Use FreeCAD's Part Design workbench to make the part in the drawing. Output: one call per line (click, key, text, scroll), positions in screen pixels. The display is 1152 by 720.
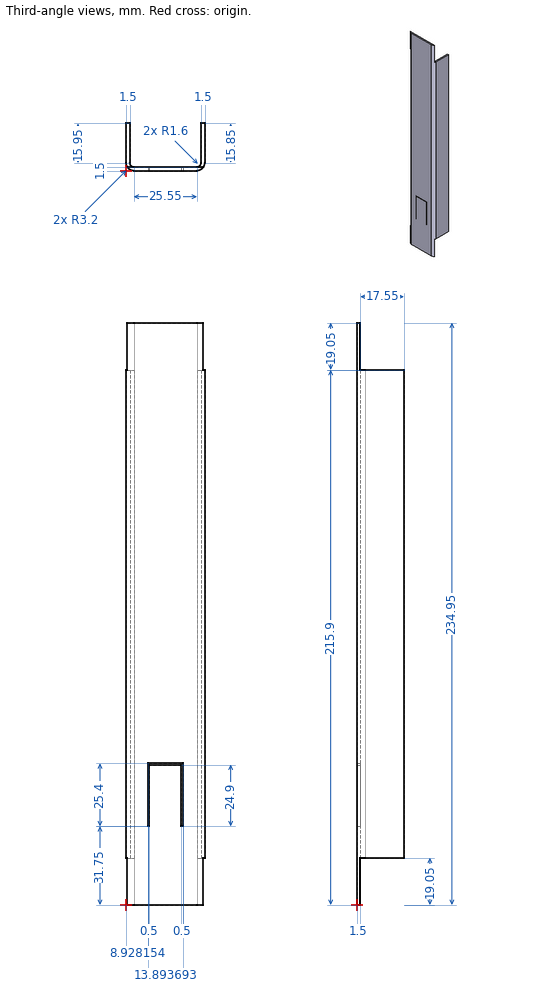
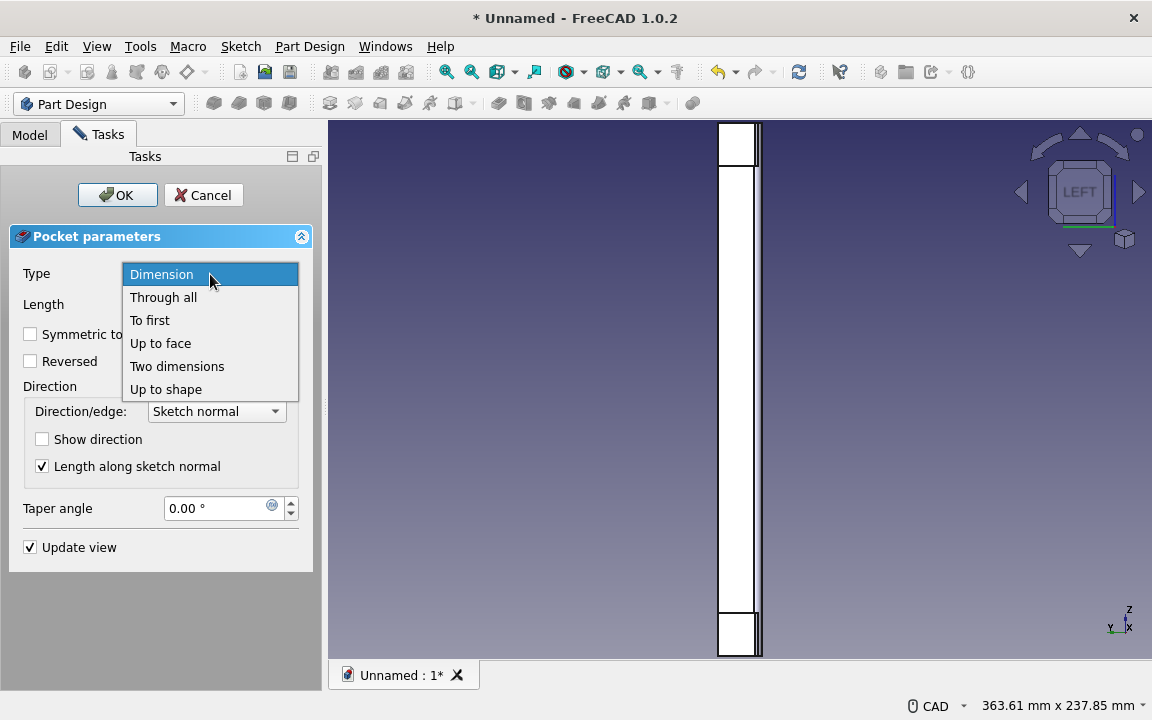
click(208, 298)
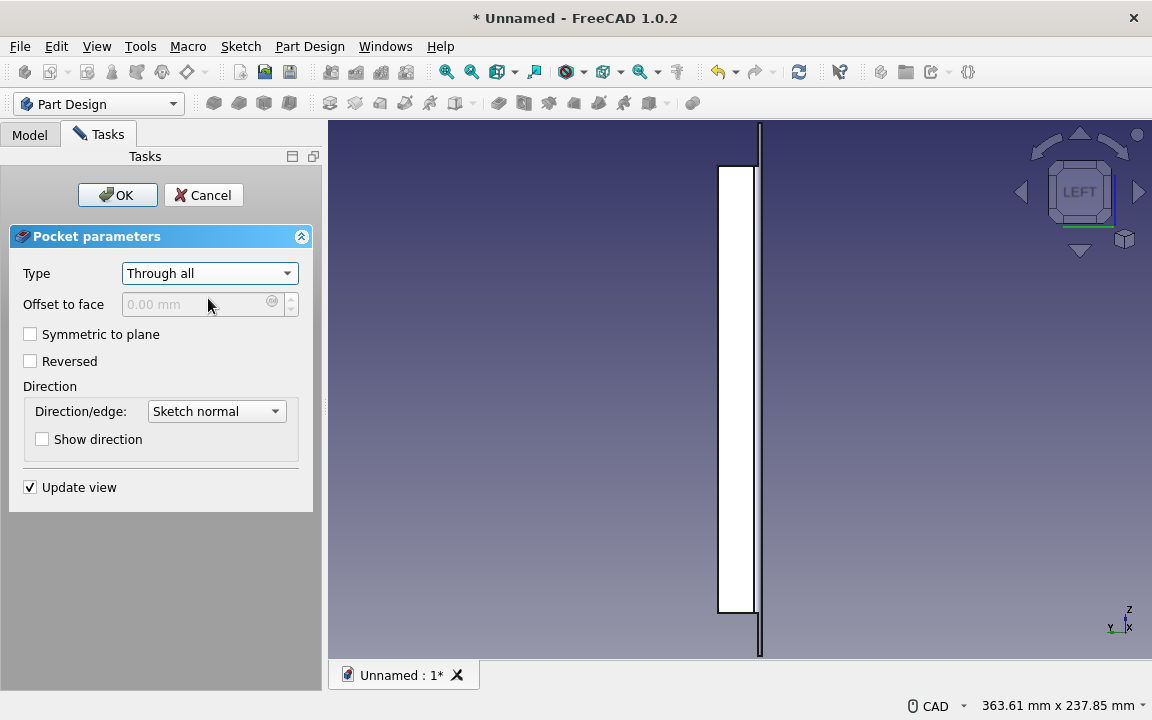
click(118, 195)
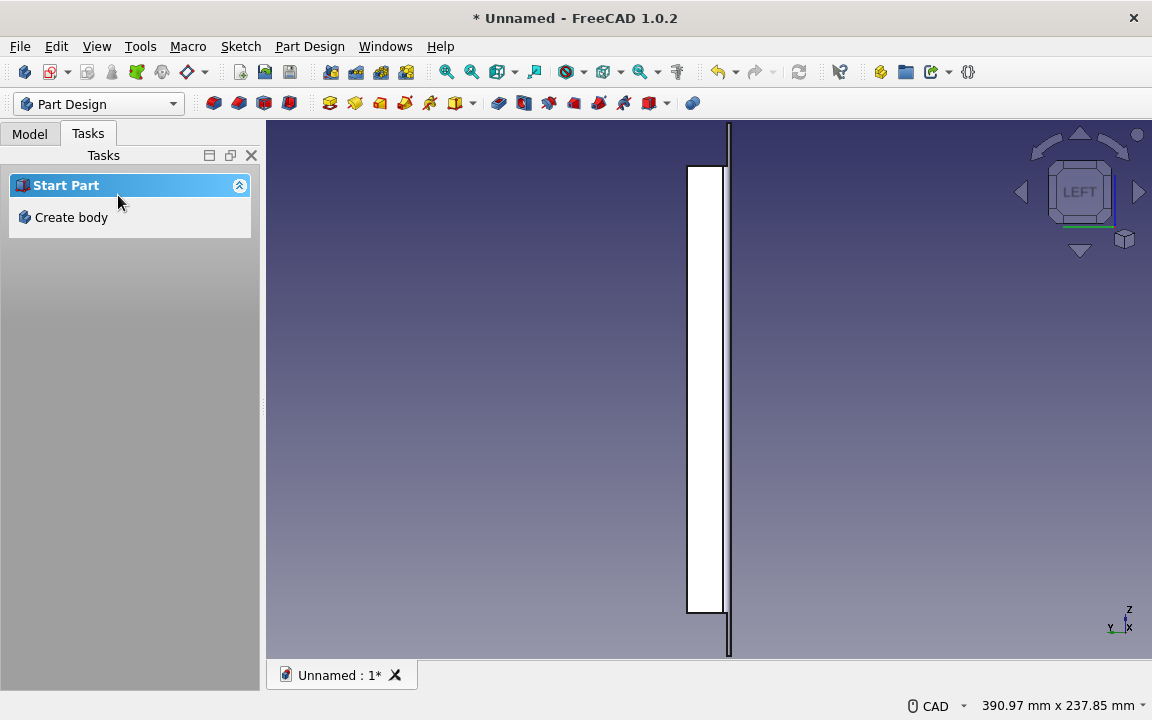
key(0)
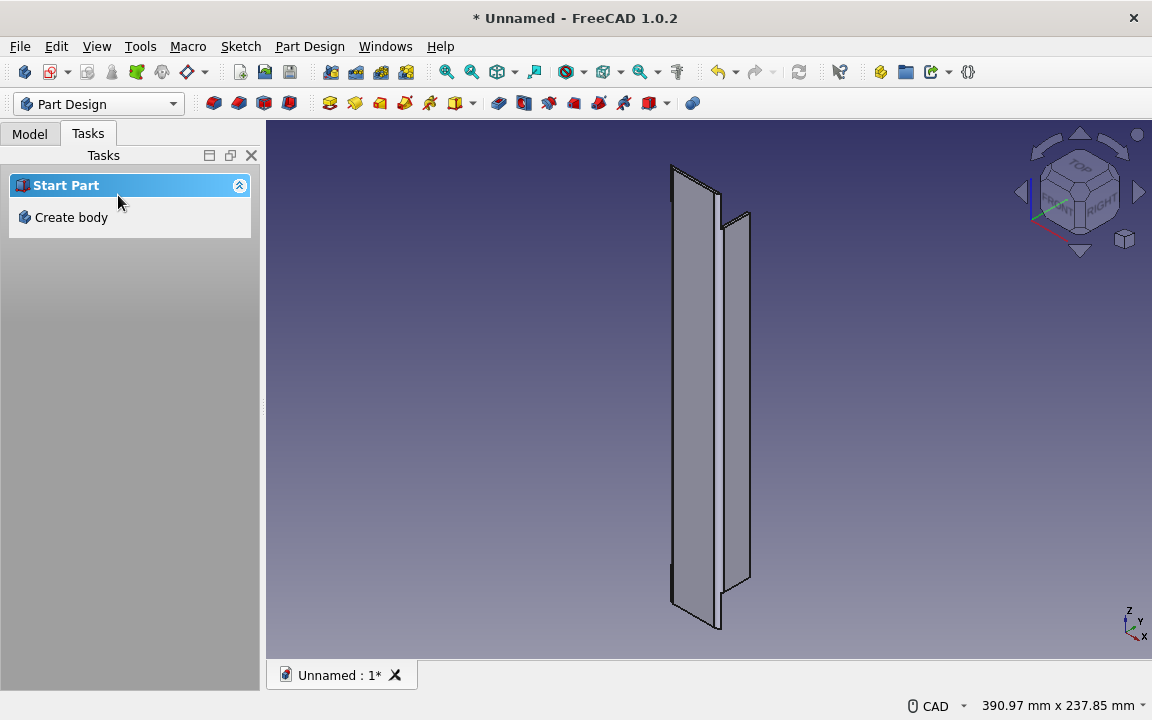
click(694, 211)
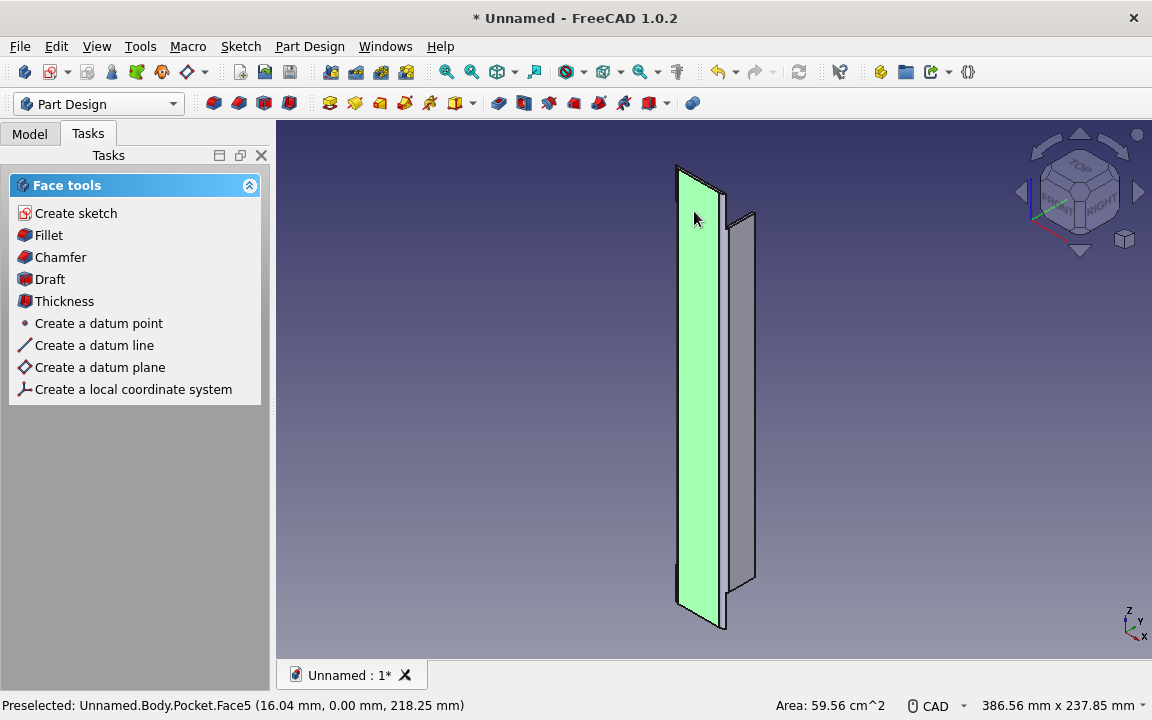
click(50, 72)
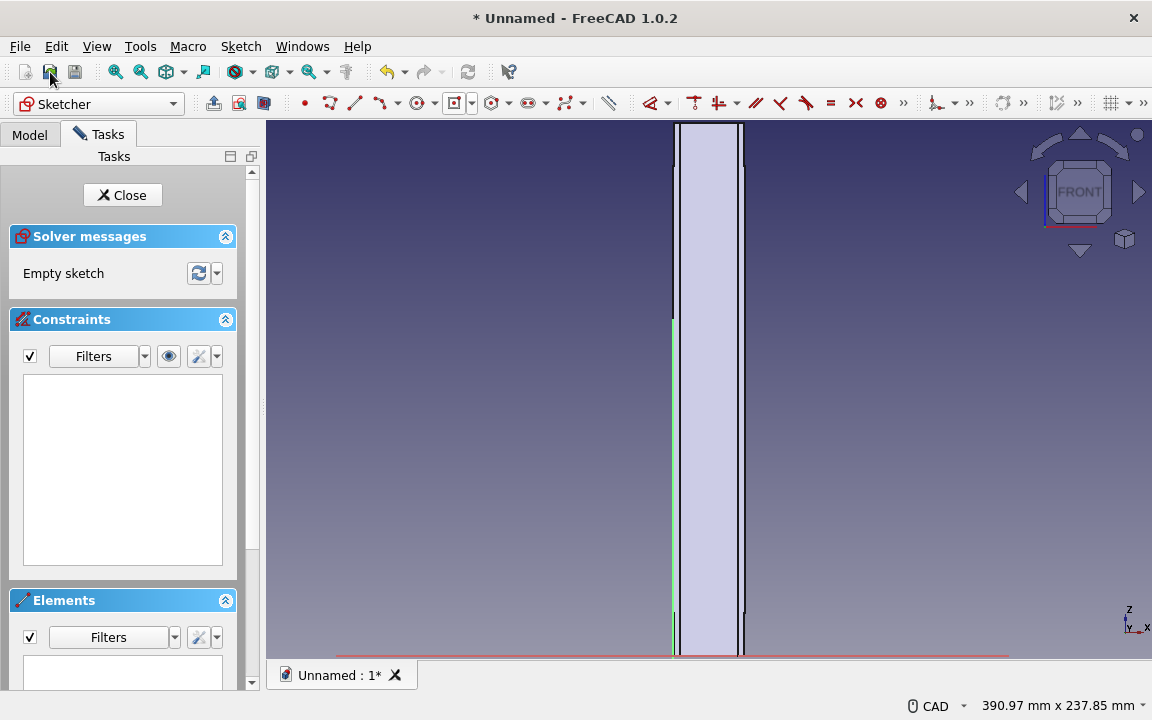
scroll(640, 390, down, 5)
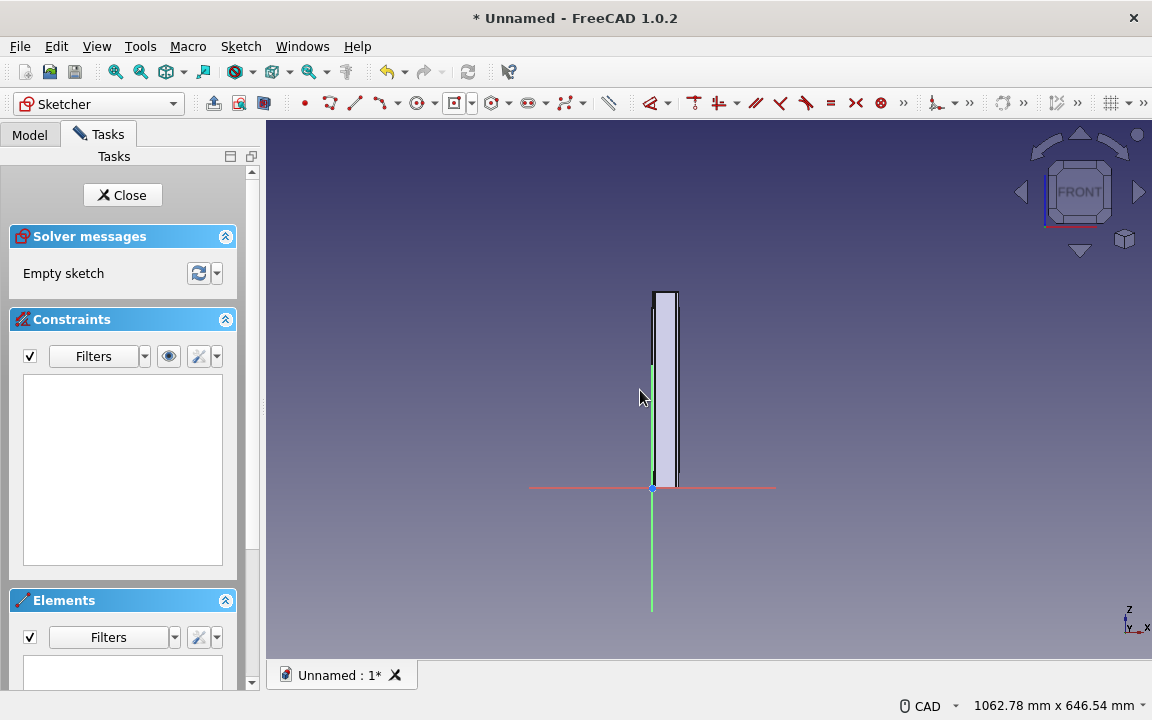
scroll(665, 476, up, 10)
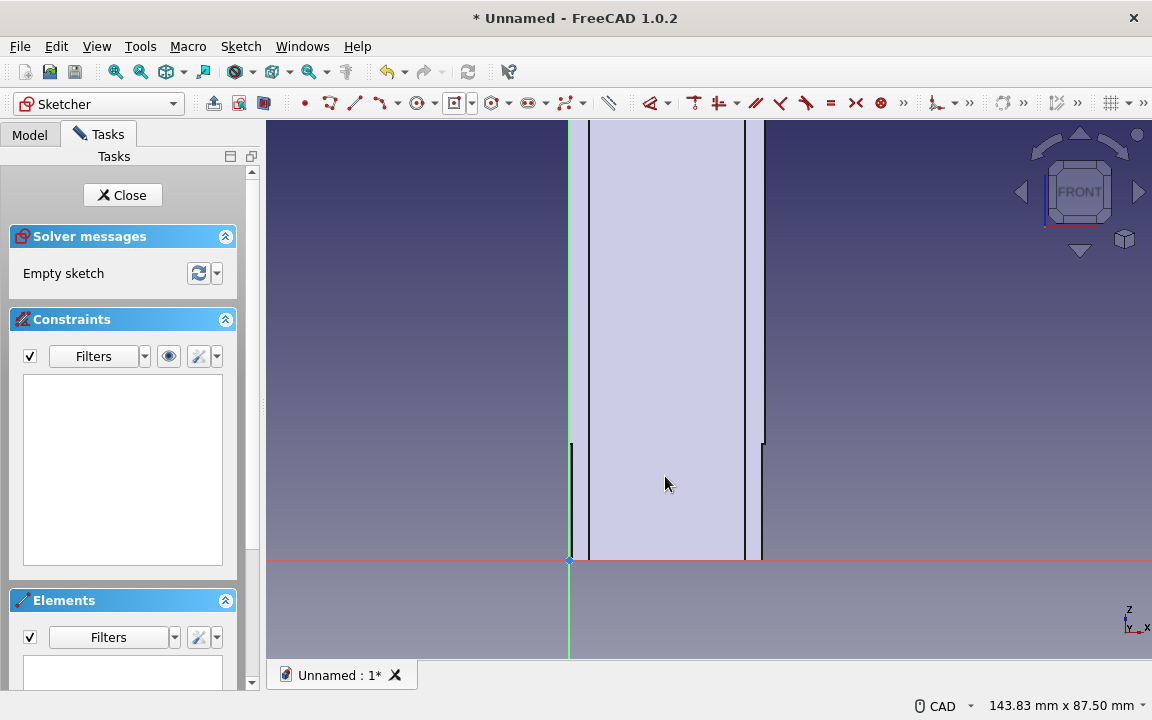
key(g)
key(m)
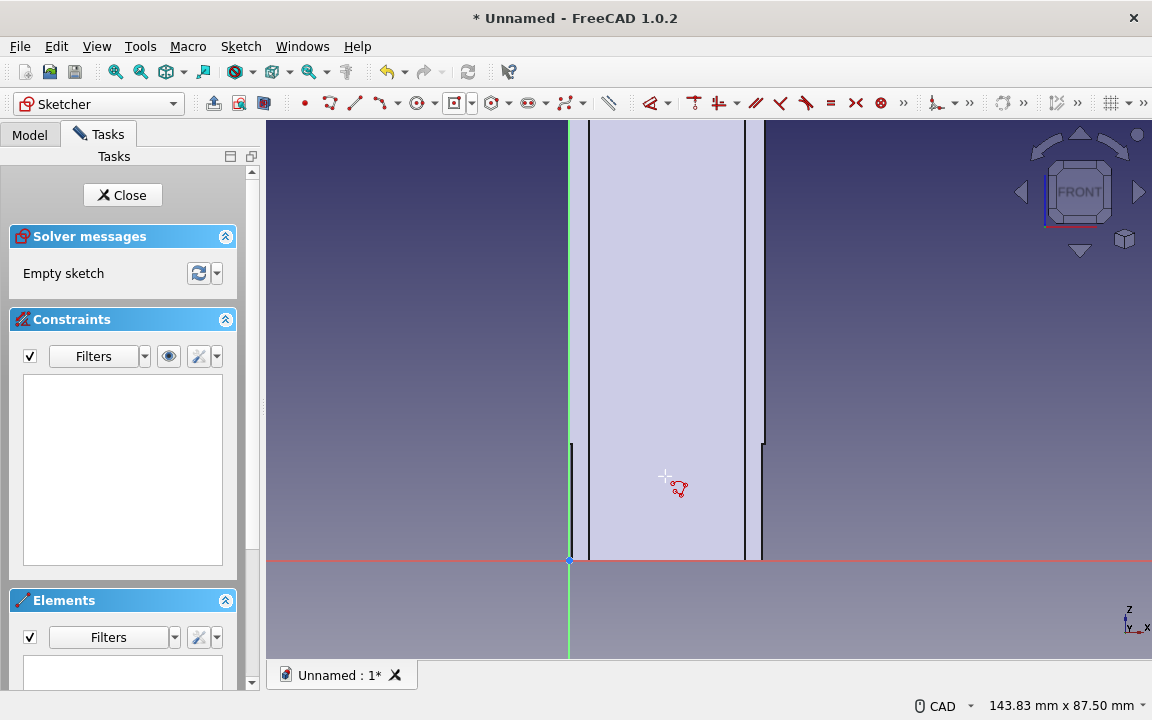
click(624, 365)
click(624, 209)
click(710, 209)
click(710, 365)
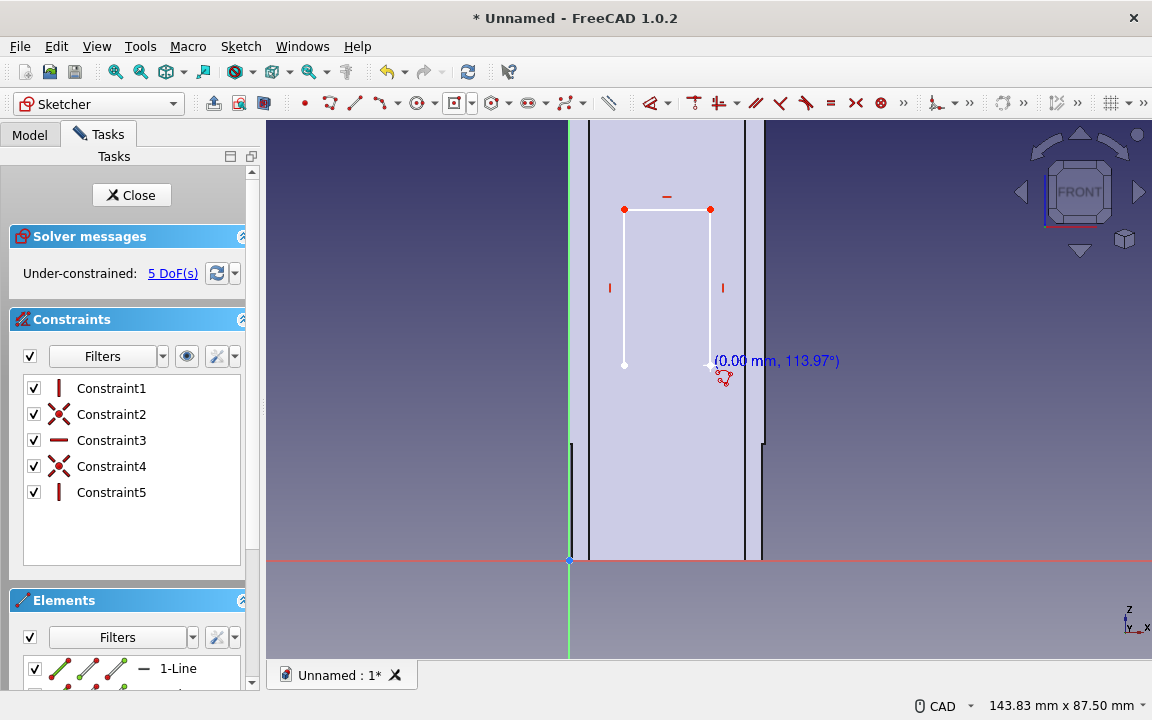
scroll(707, 365, up, 9)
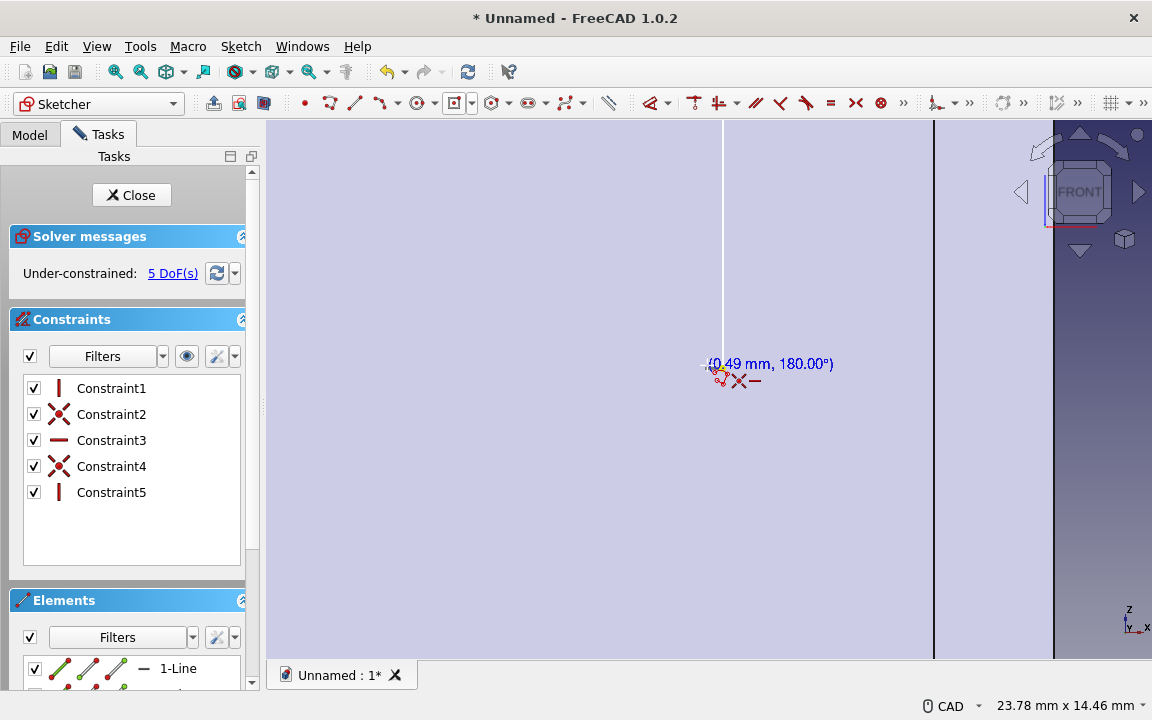
click(702, 363)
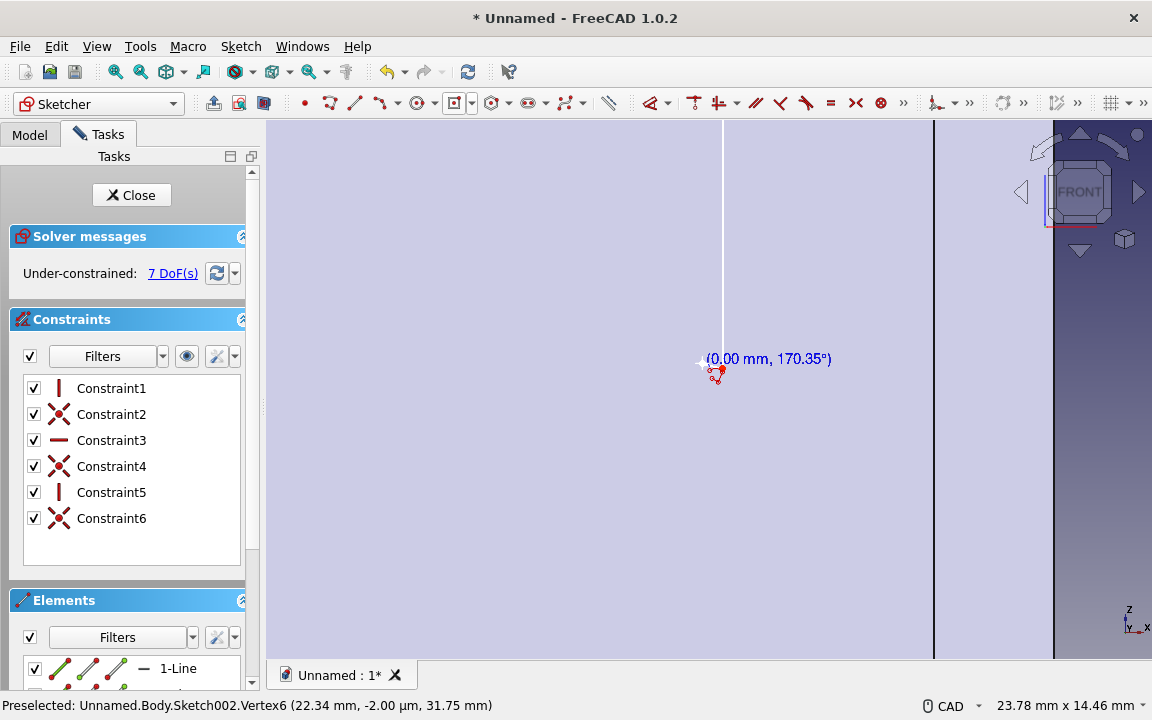
scroll(709, 371, down, 9)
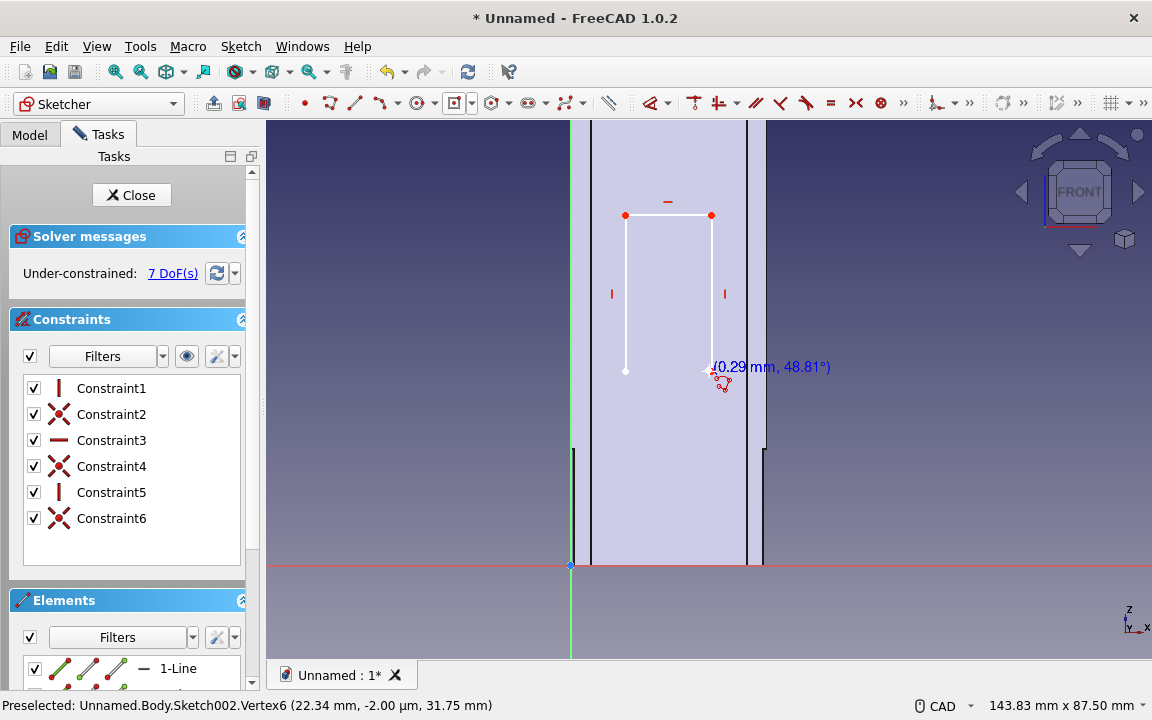
scroll(708, 217, up, 9)